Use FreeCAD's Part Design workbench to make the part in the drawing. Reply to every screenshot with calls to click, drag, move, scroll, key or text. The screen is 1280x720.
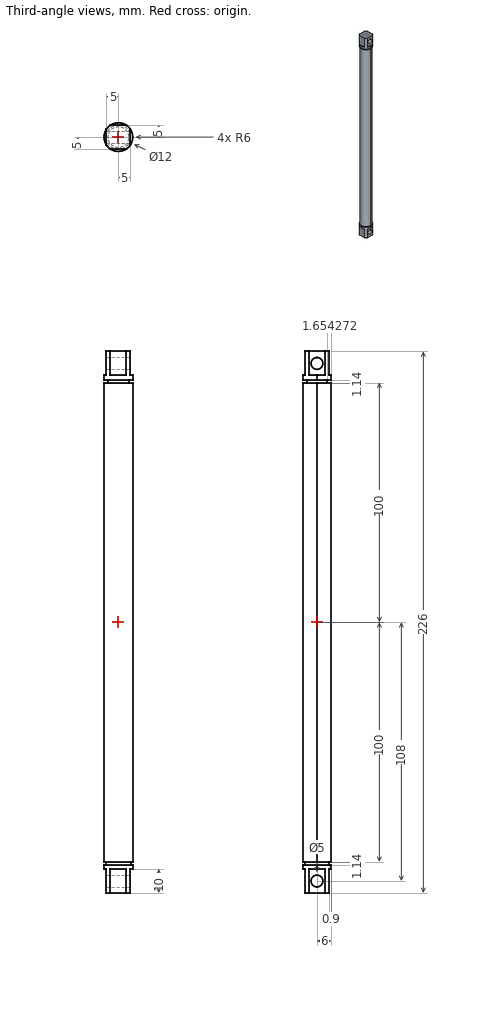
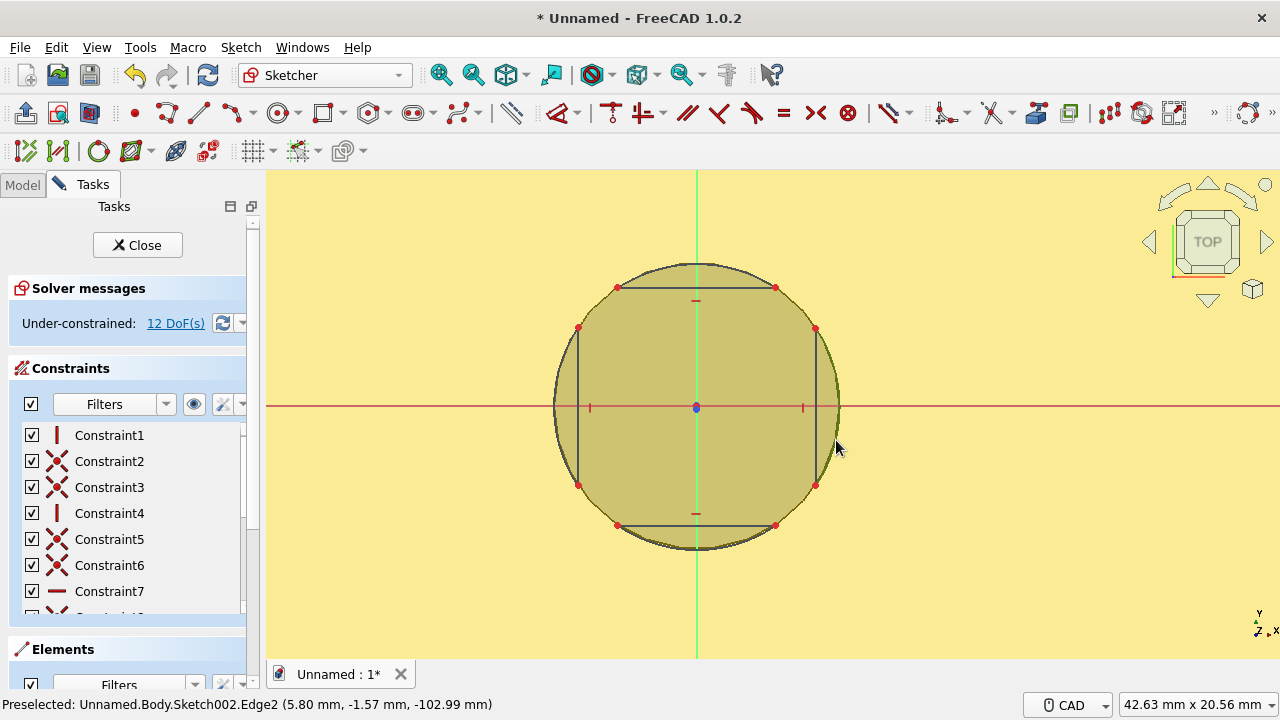
click(663, 546)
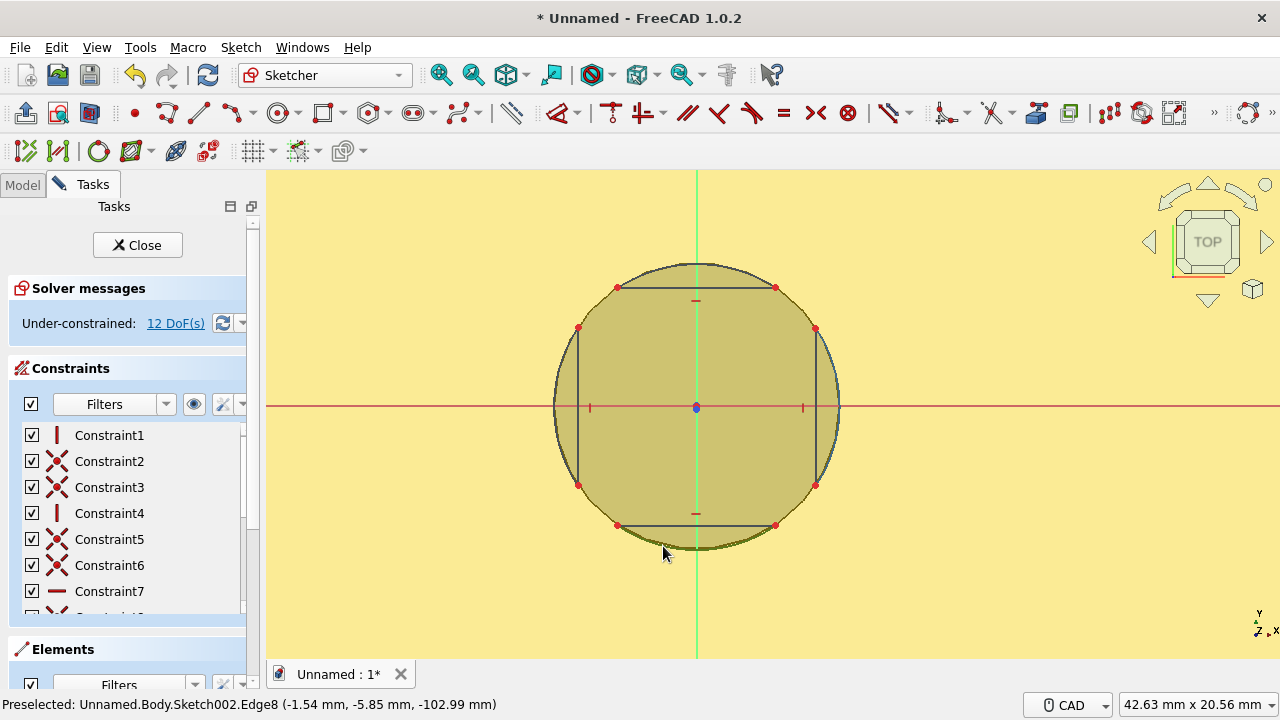
key(c)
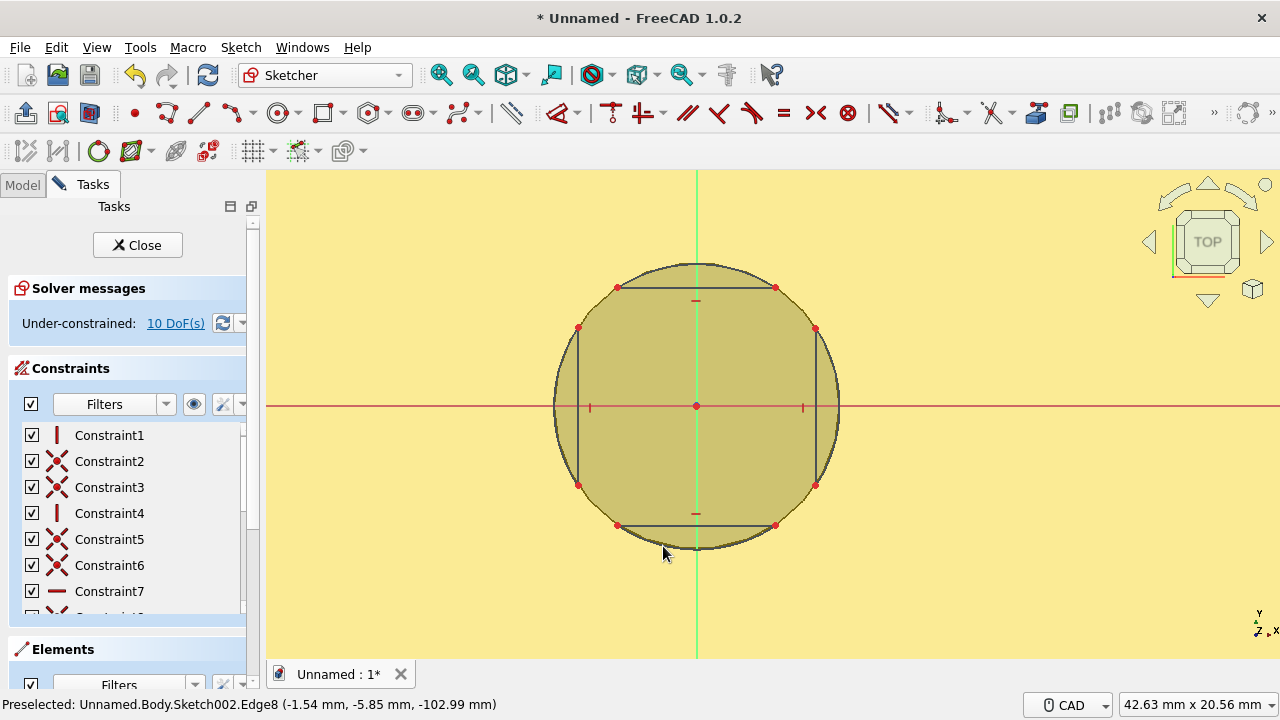
drag(687, 396, 707, 417)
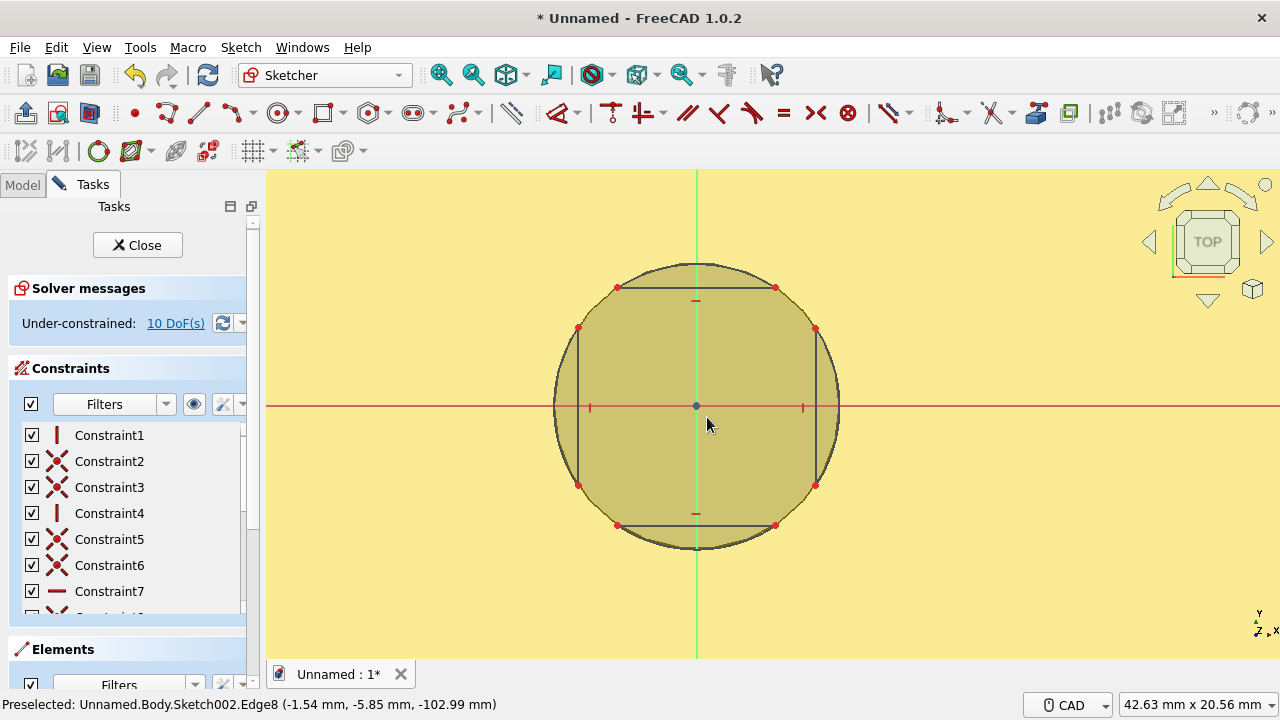
click(612, 114)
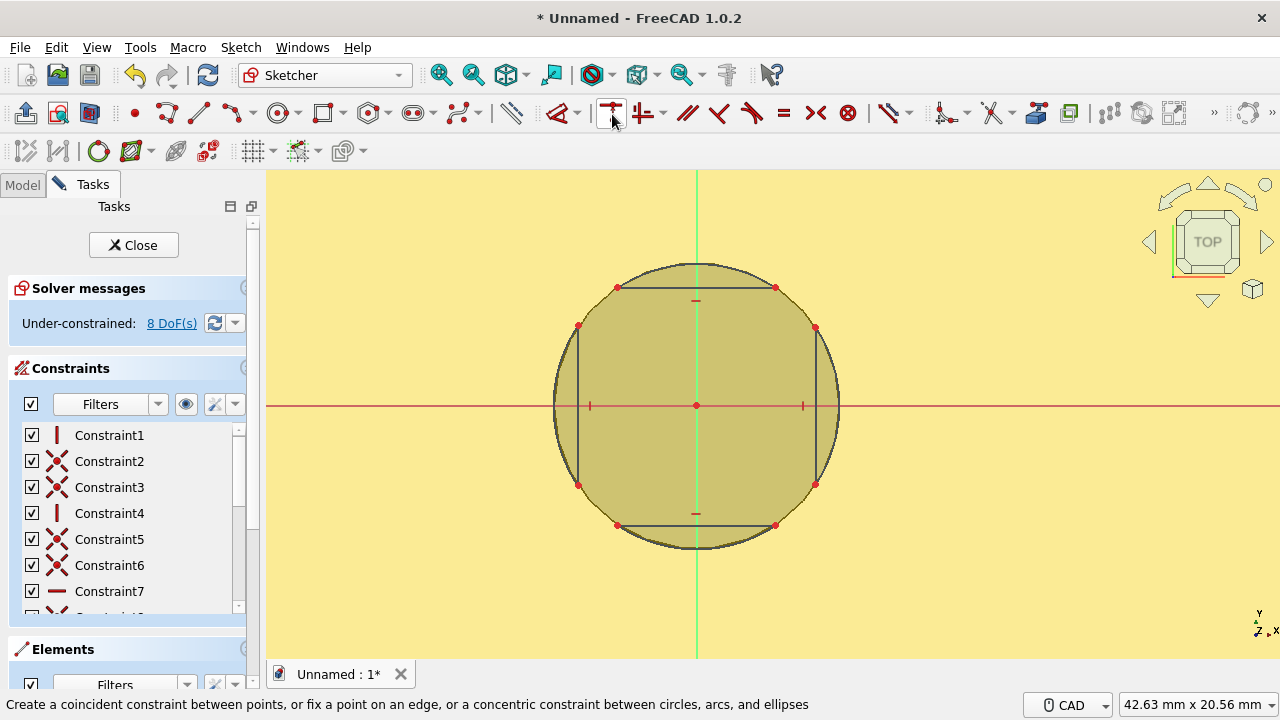
click(835, 439)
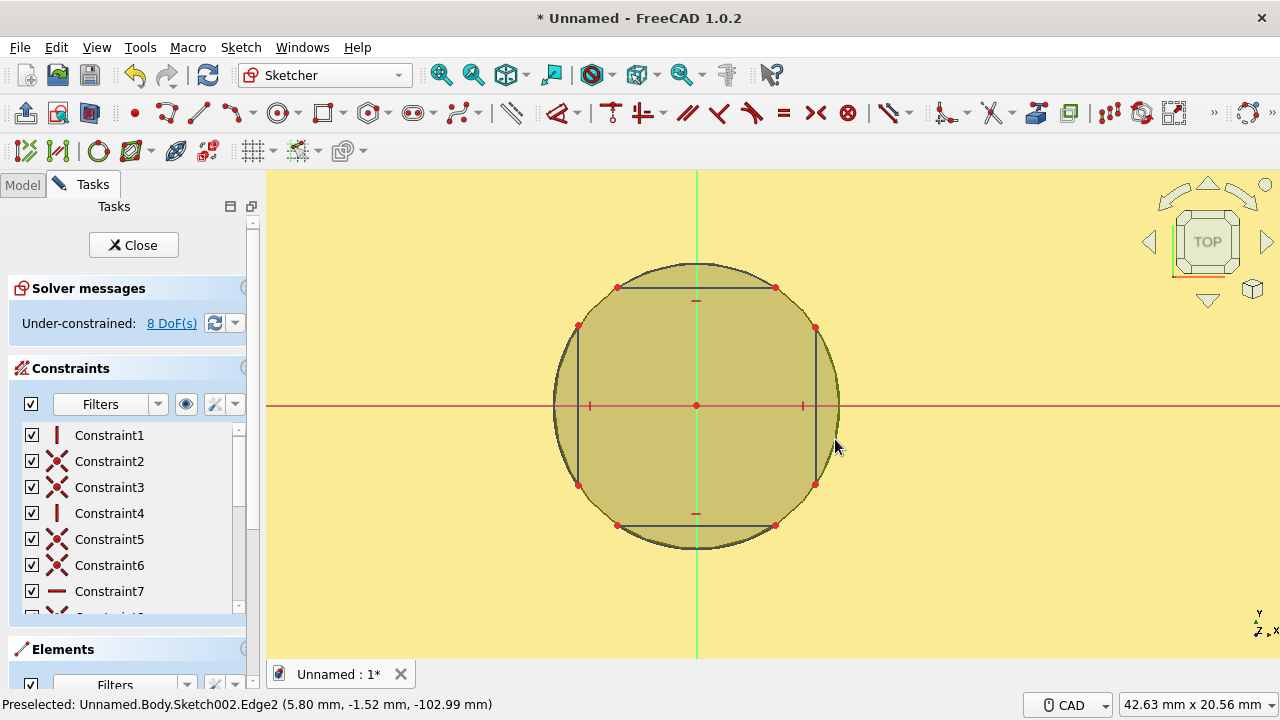
click(558, 372)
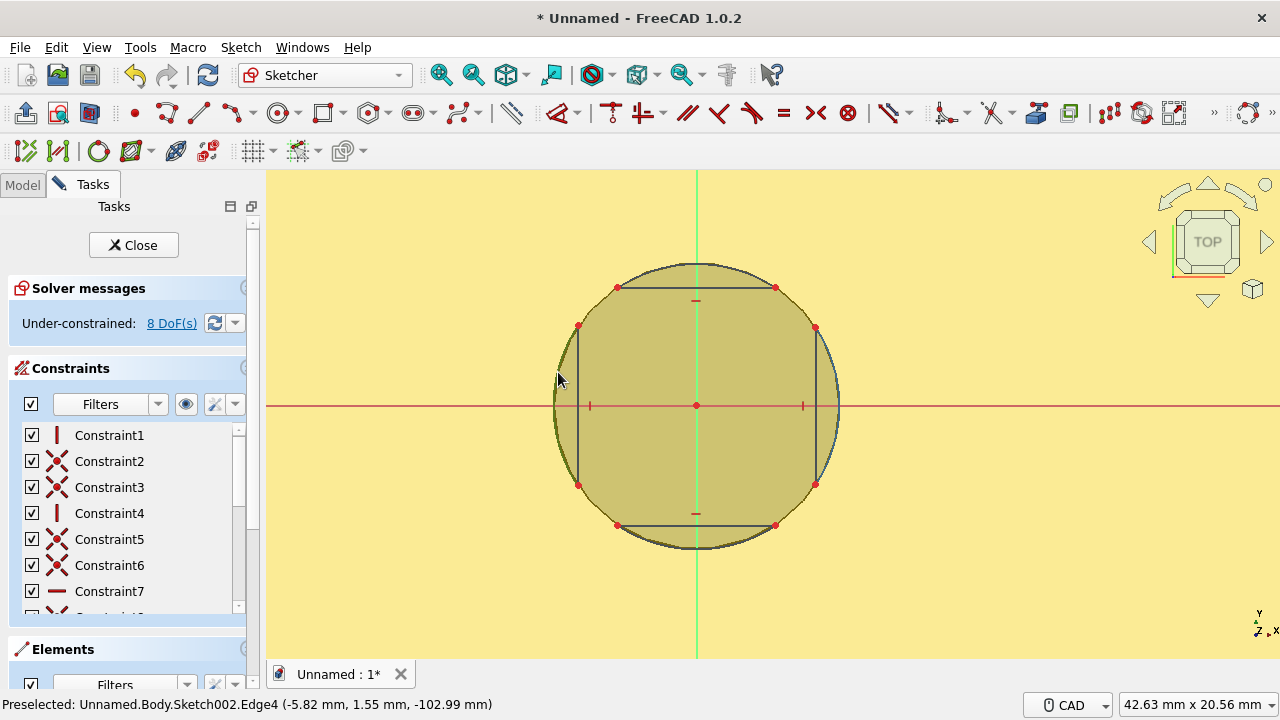
click(730, 268)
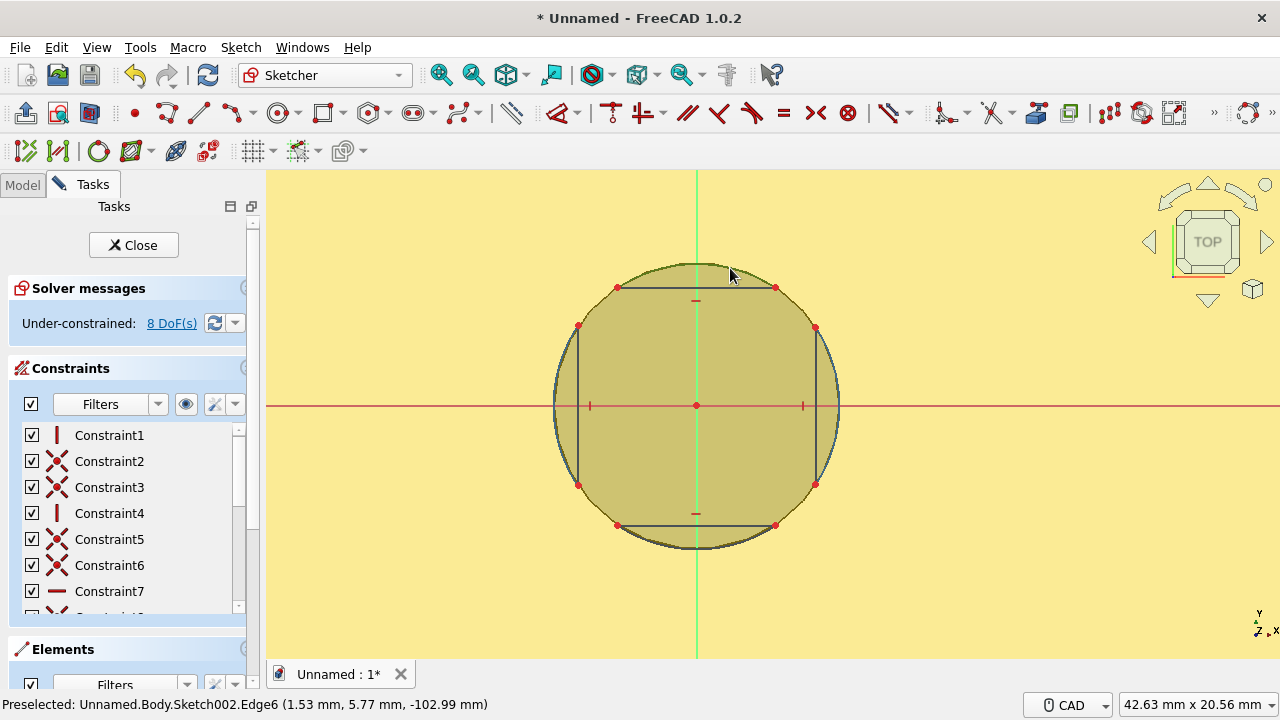
click(664, 545)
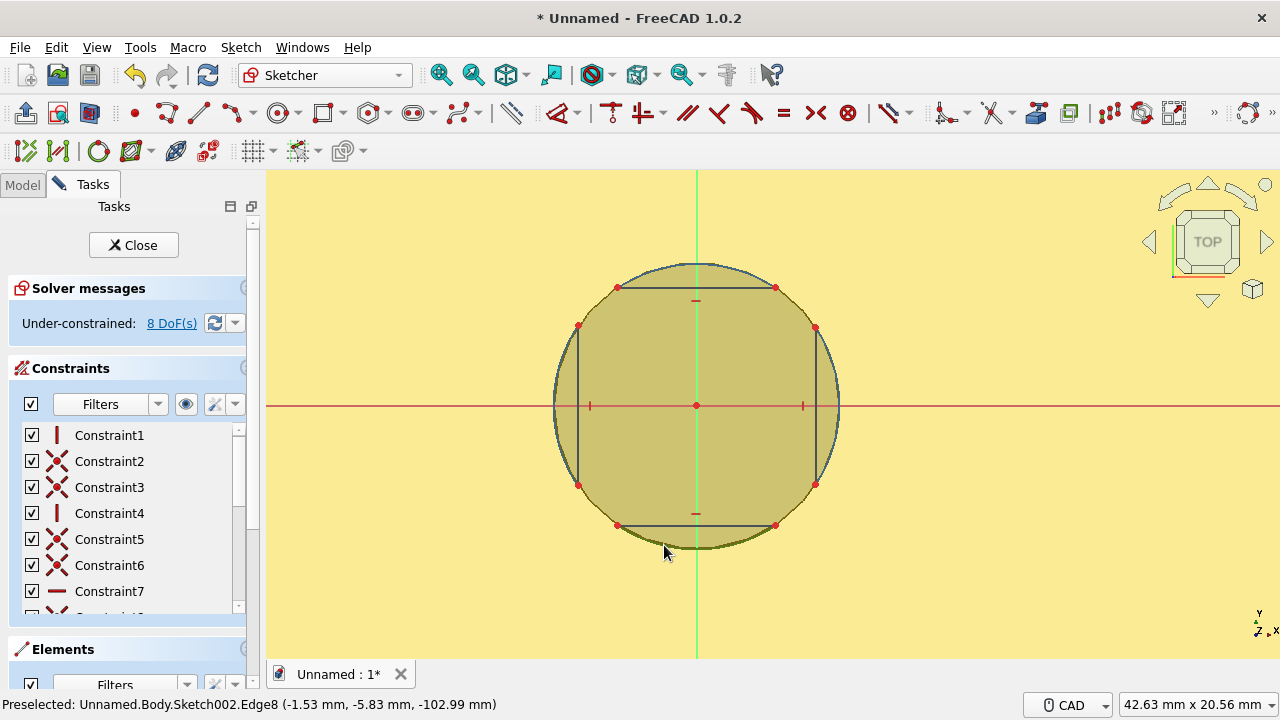
click(784, 114)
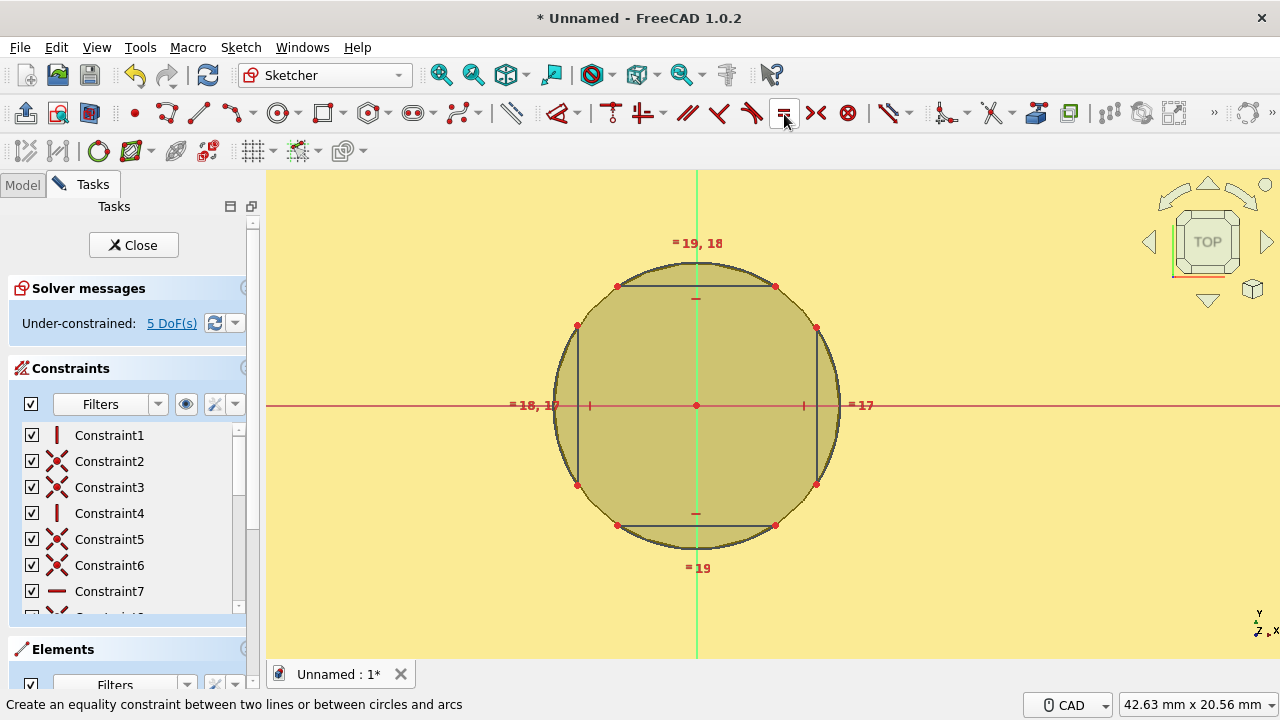
click(558, 114)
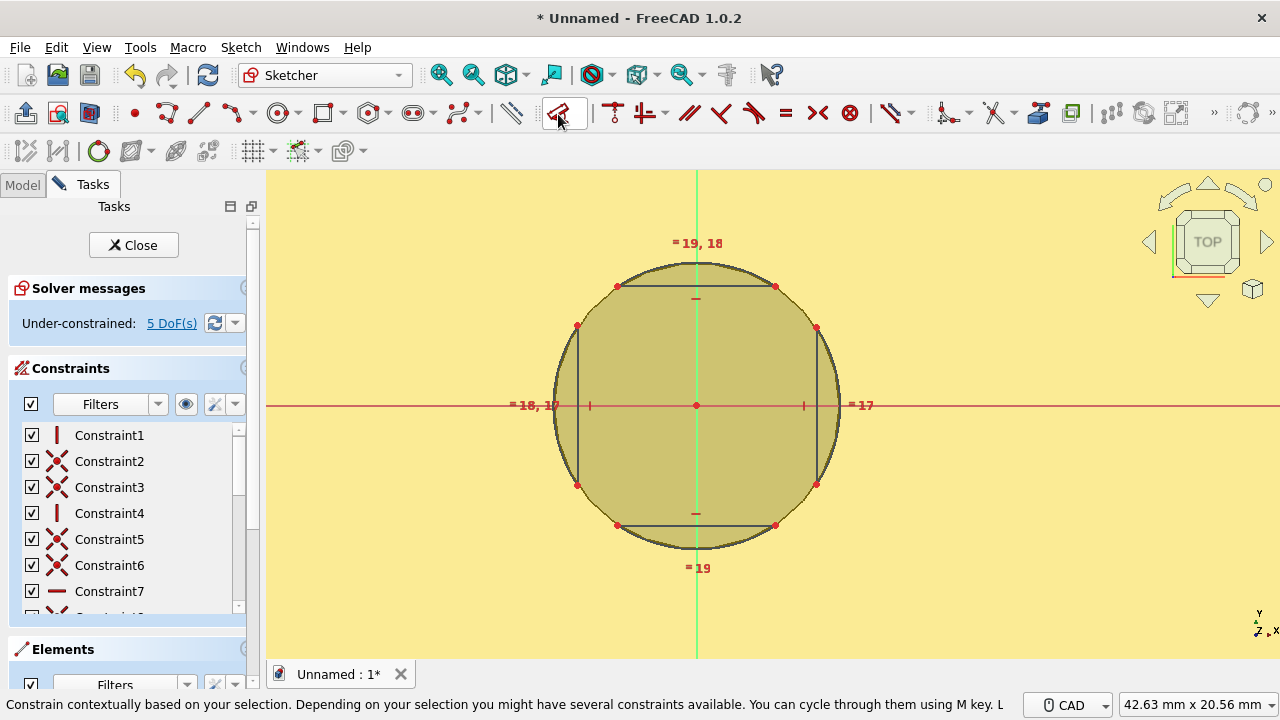
click(836, 439)
click(867, 446)